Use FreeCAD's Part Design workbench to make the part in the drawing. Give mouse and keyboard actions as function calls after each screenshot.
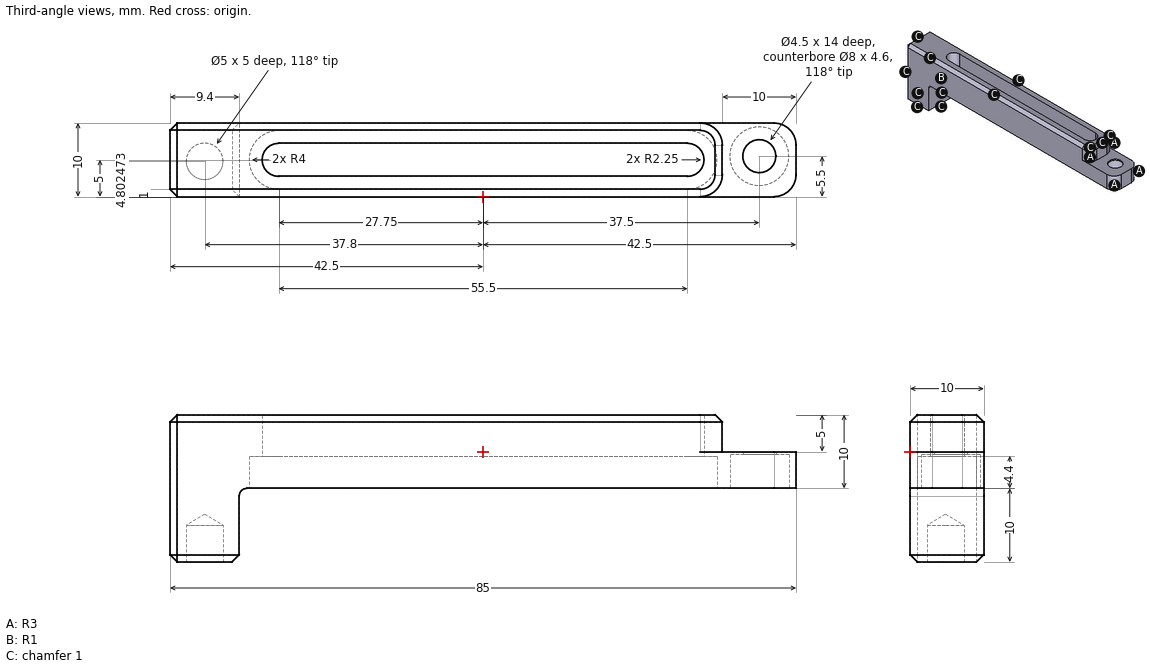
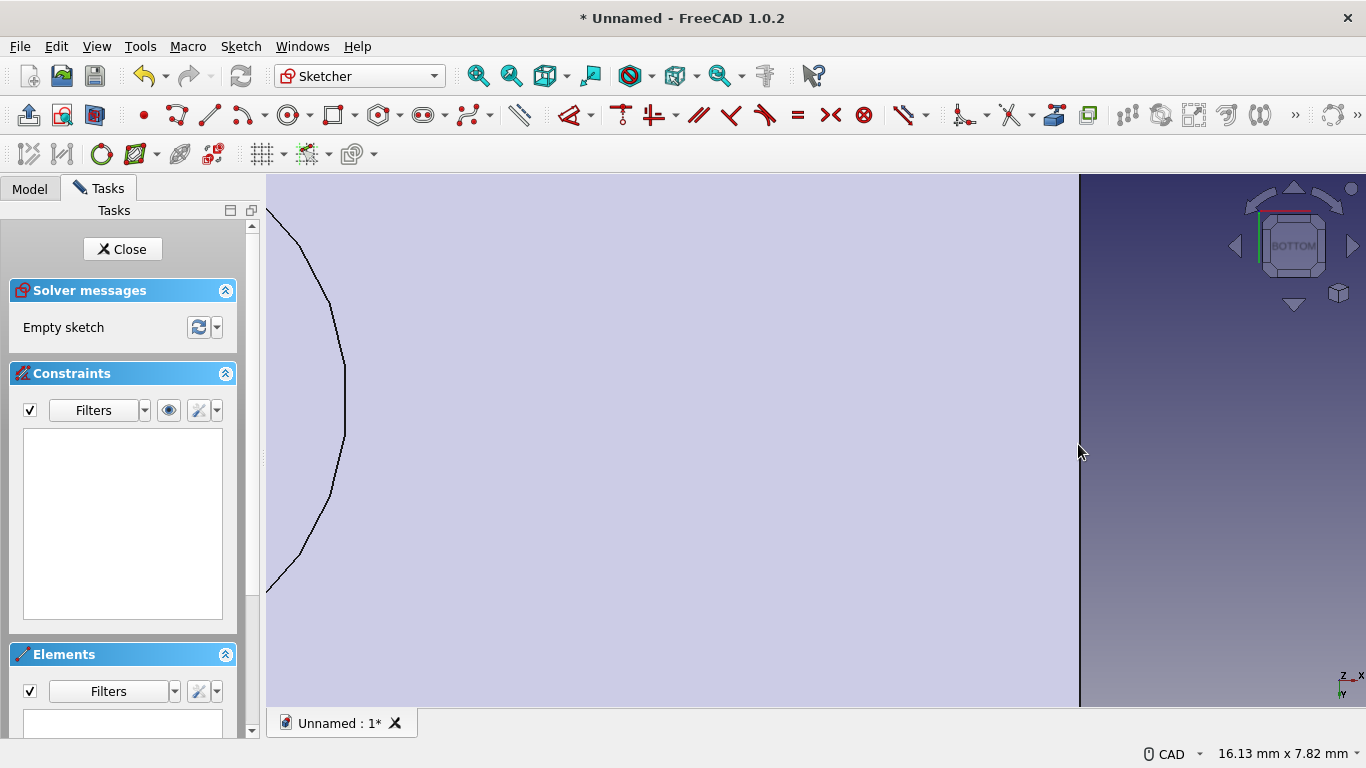
key(g)
key(c)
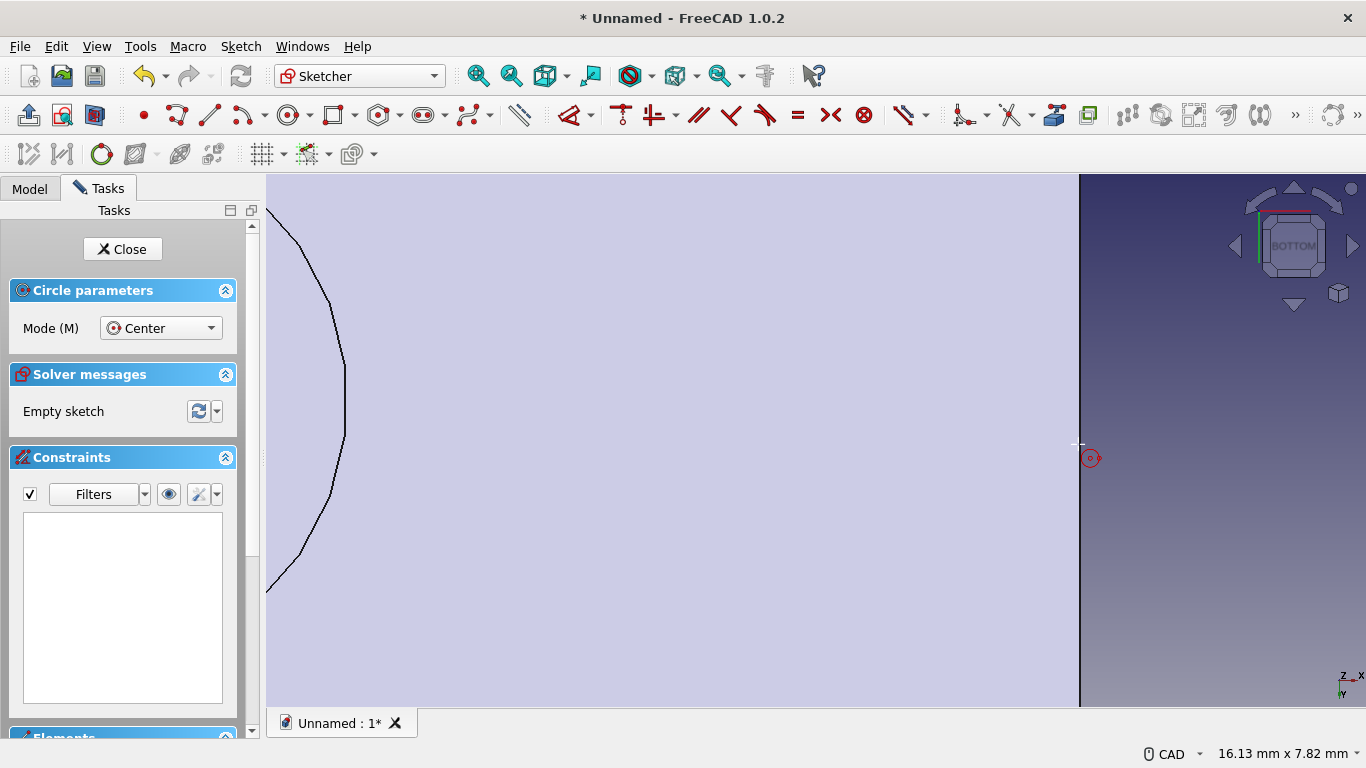
click(739, 434)
click(848, 326)
key(Escape)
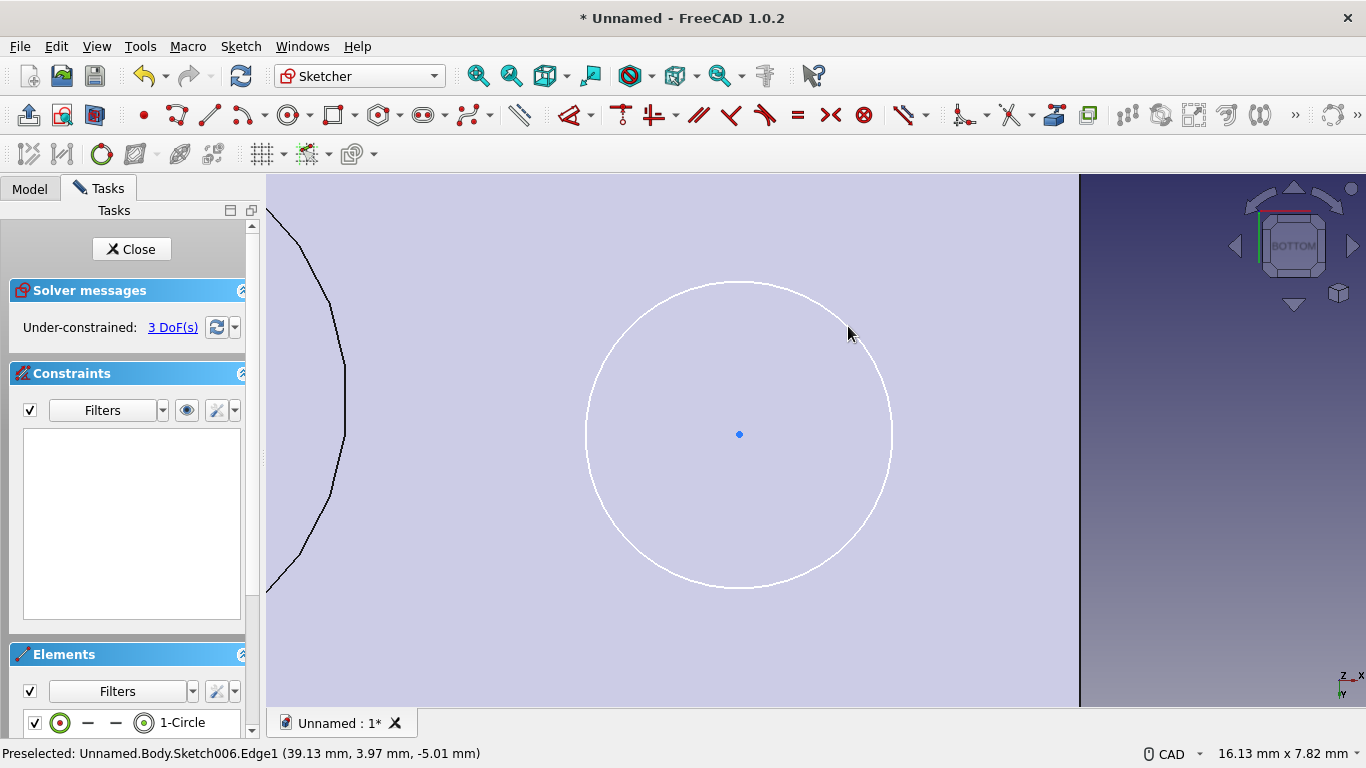
click(568, 116)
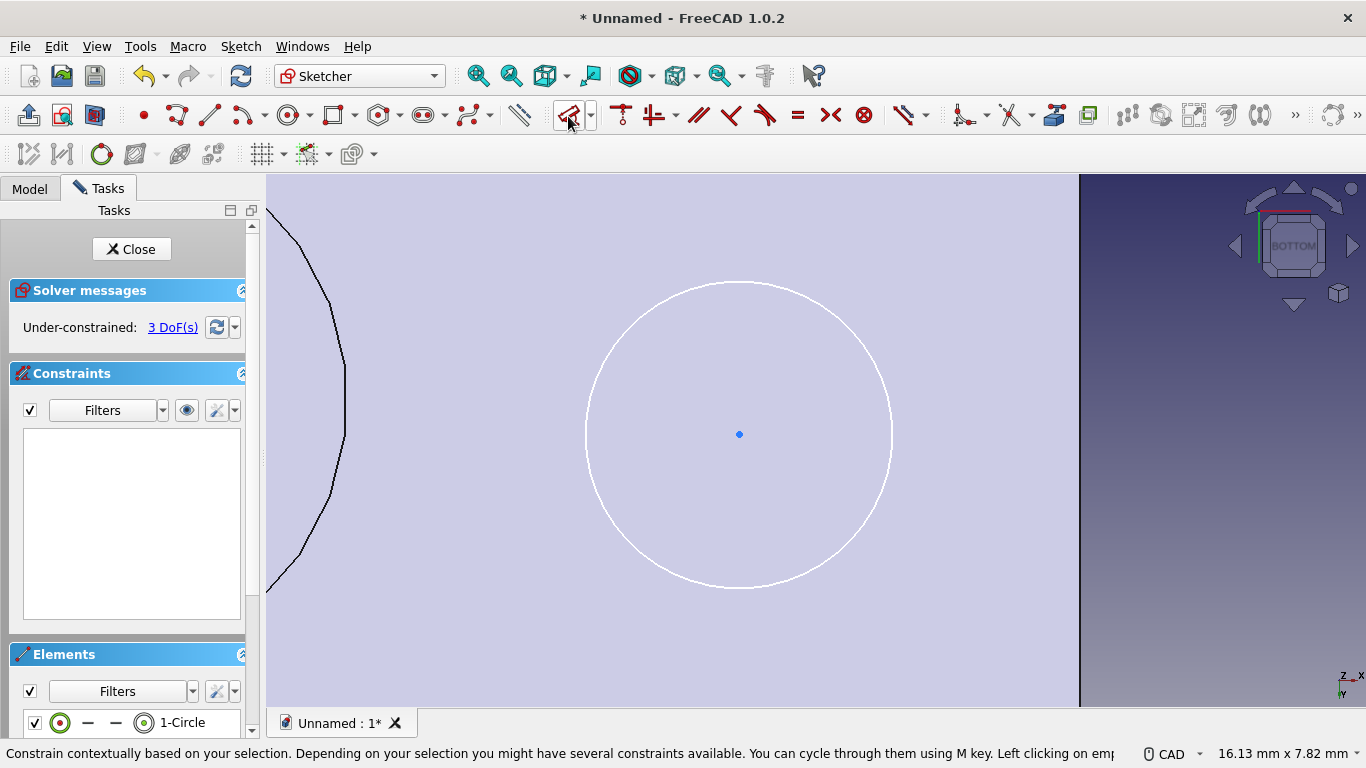
click(847, 326)
click(870, 303)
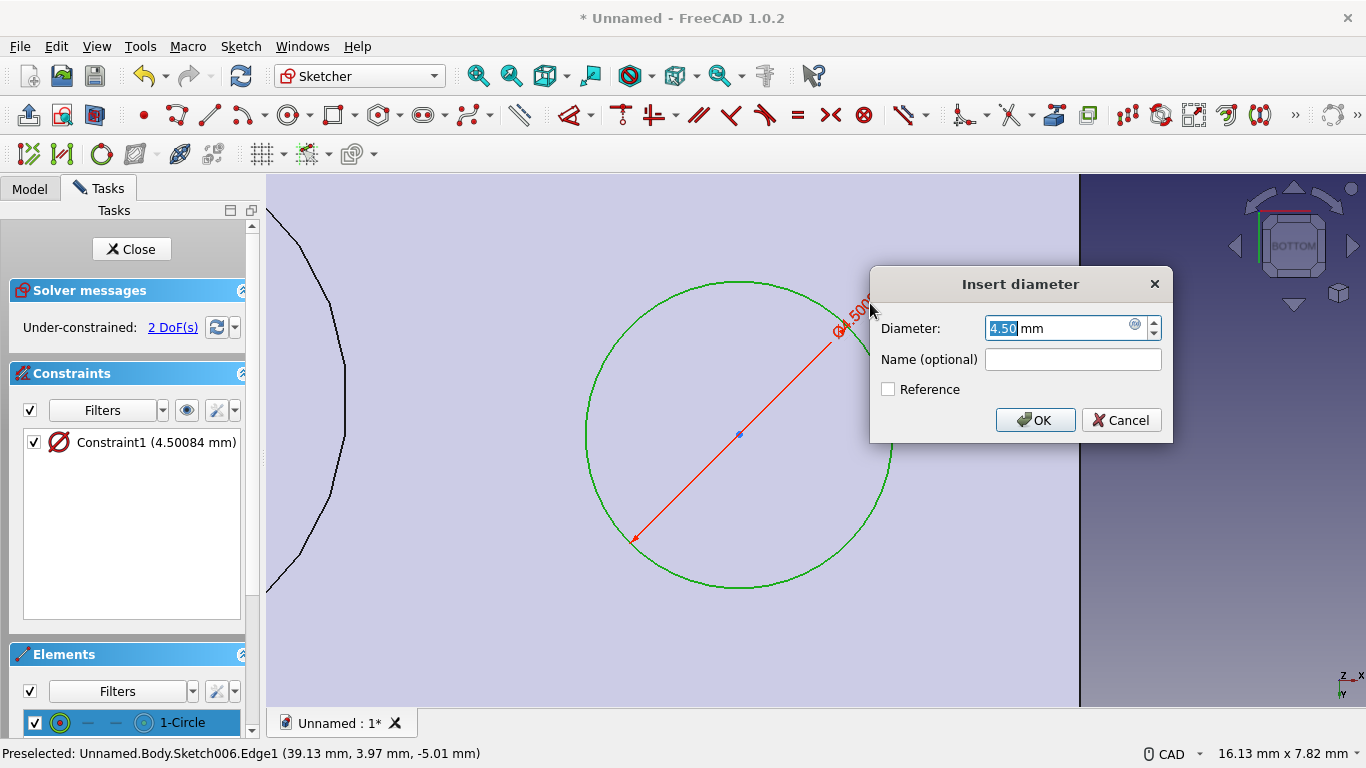
text(4.5)
key(Return)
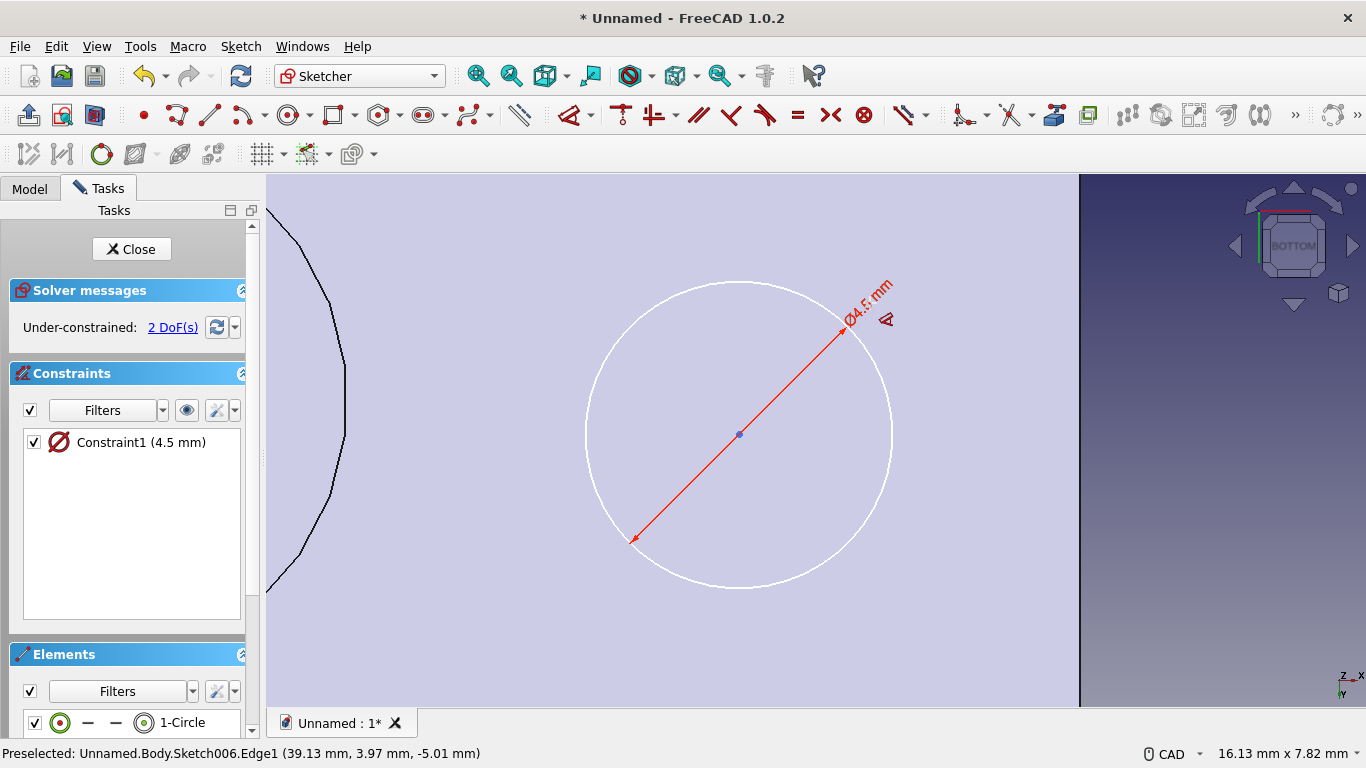
click(739, 435)
click(773, 319)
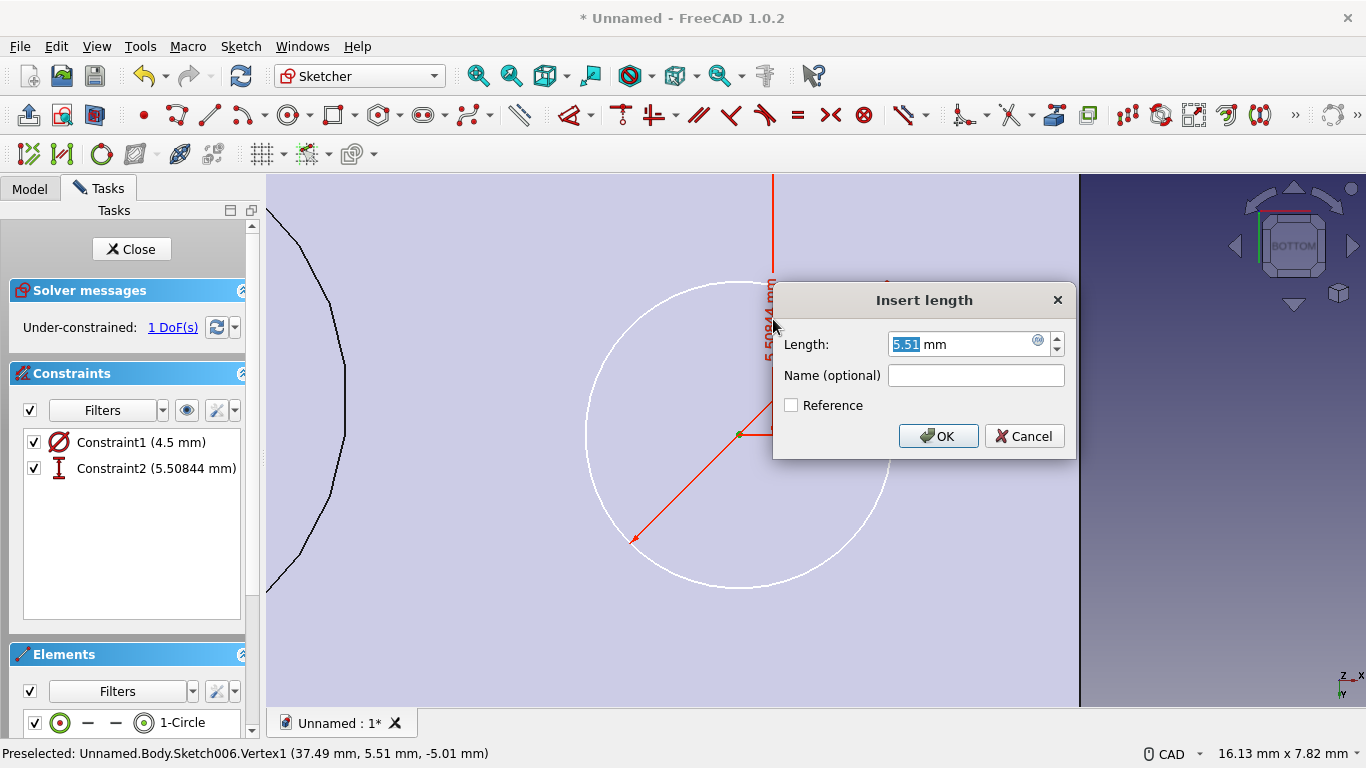
text(5.5)
key(Return)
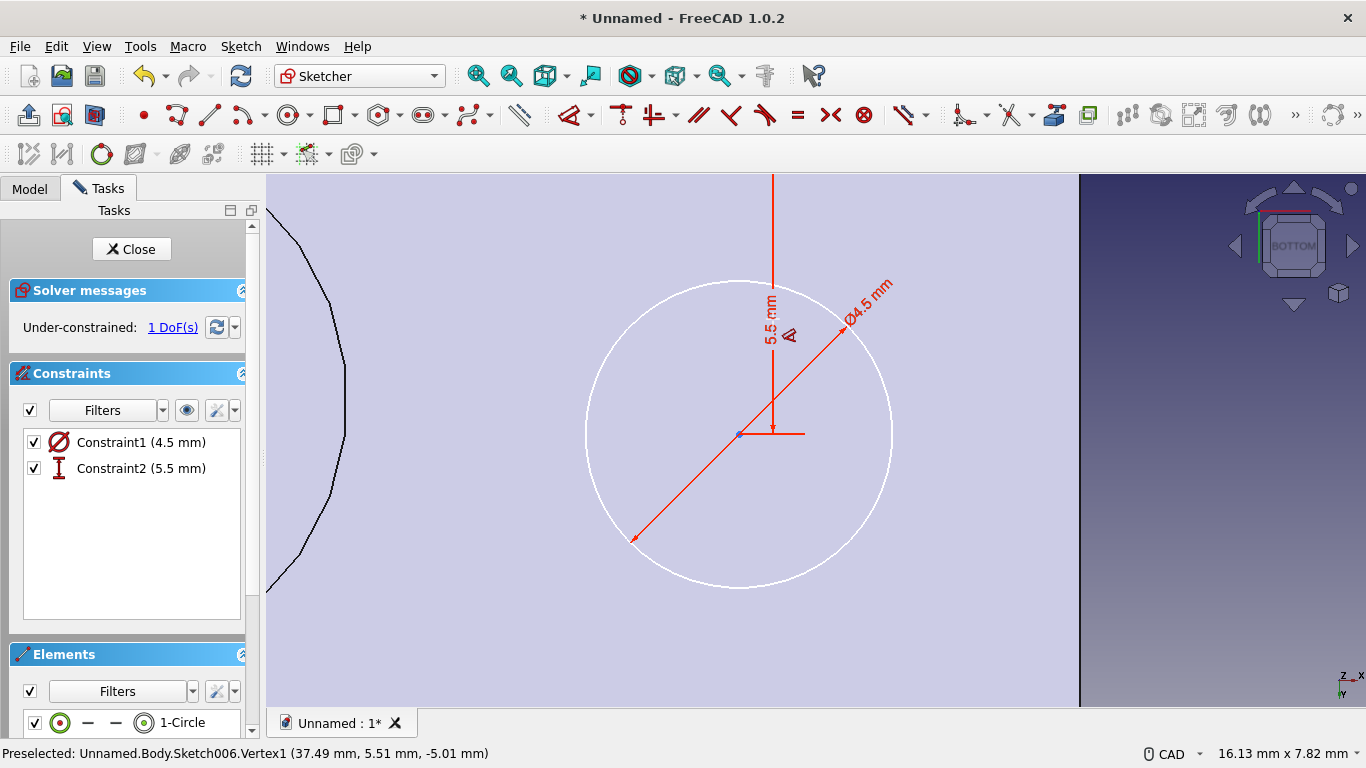
click(739, 434)
click(517, 468)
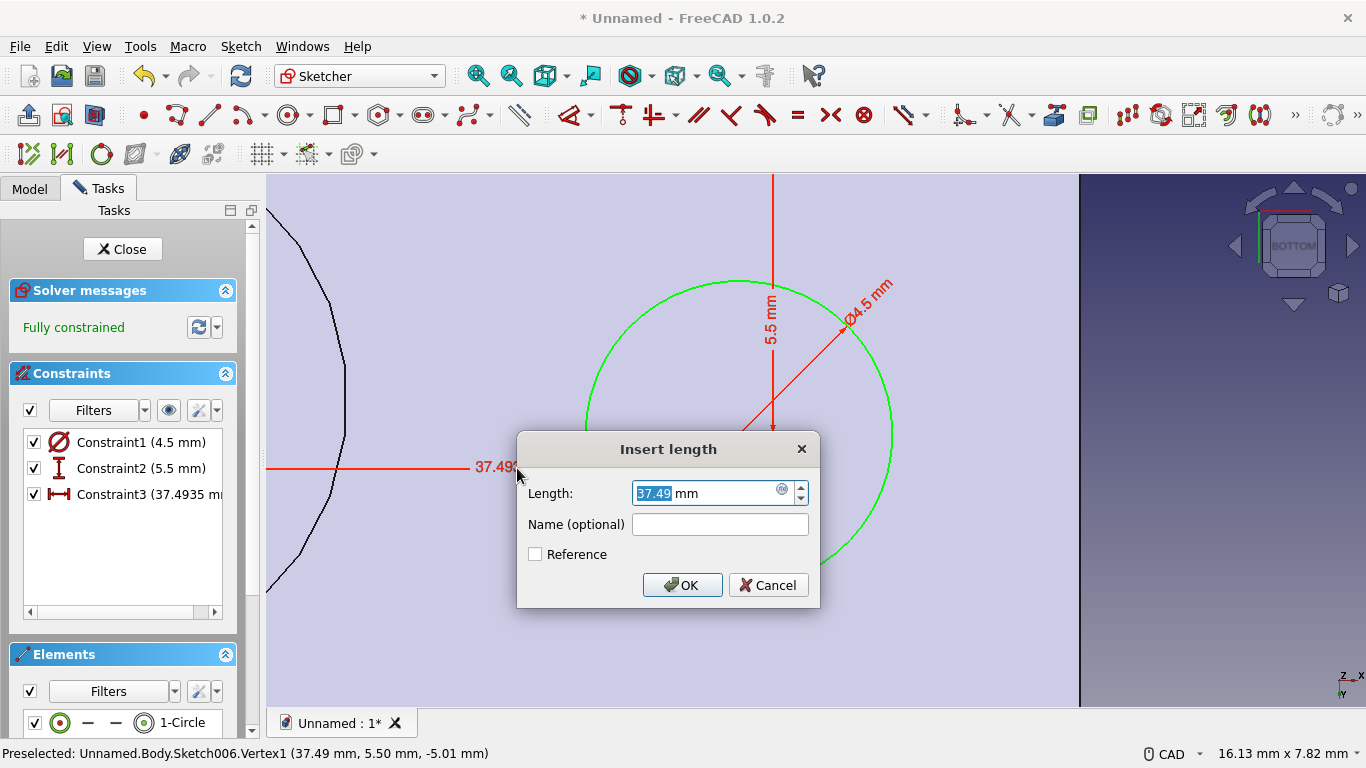
text(37.5)
key(Return)
key(Escape)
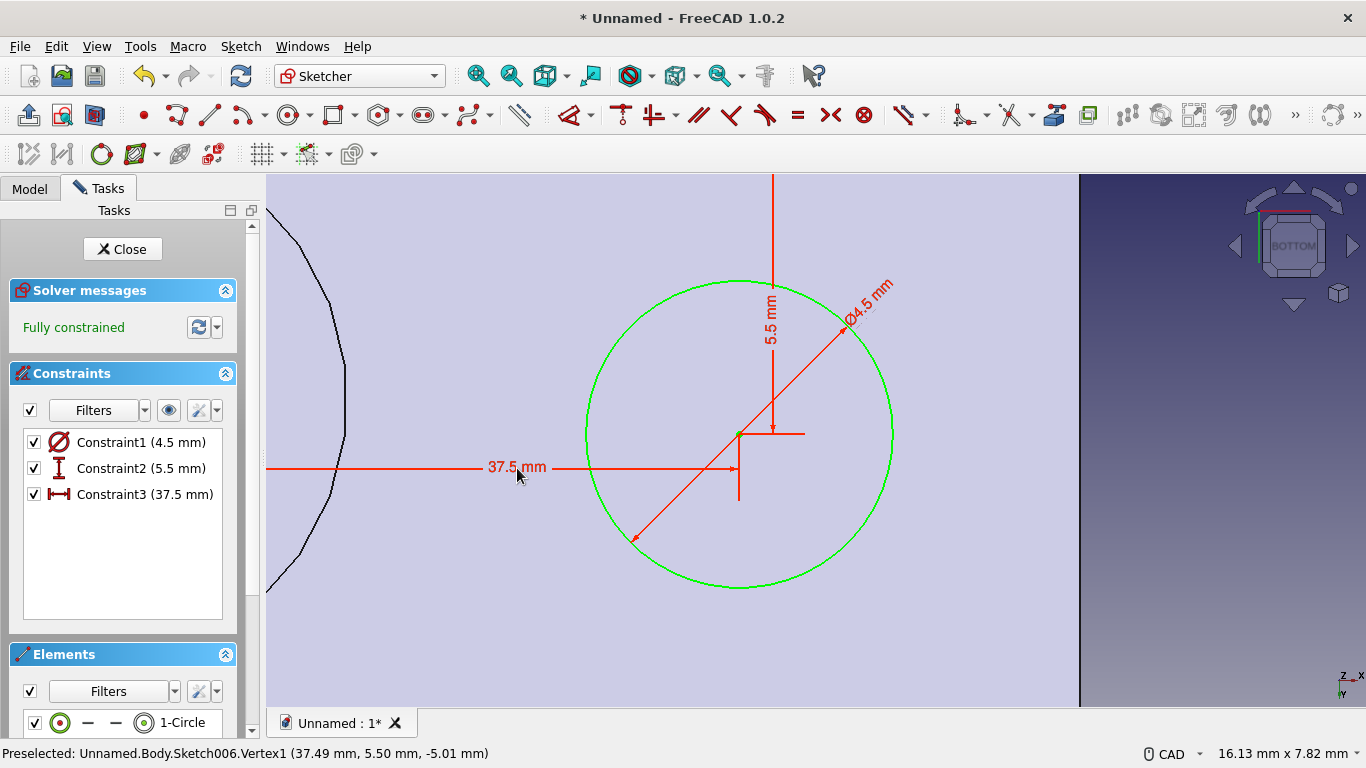
click(123, 249)